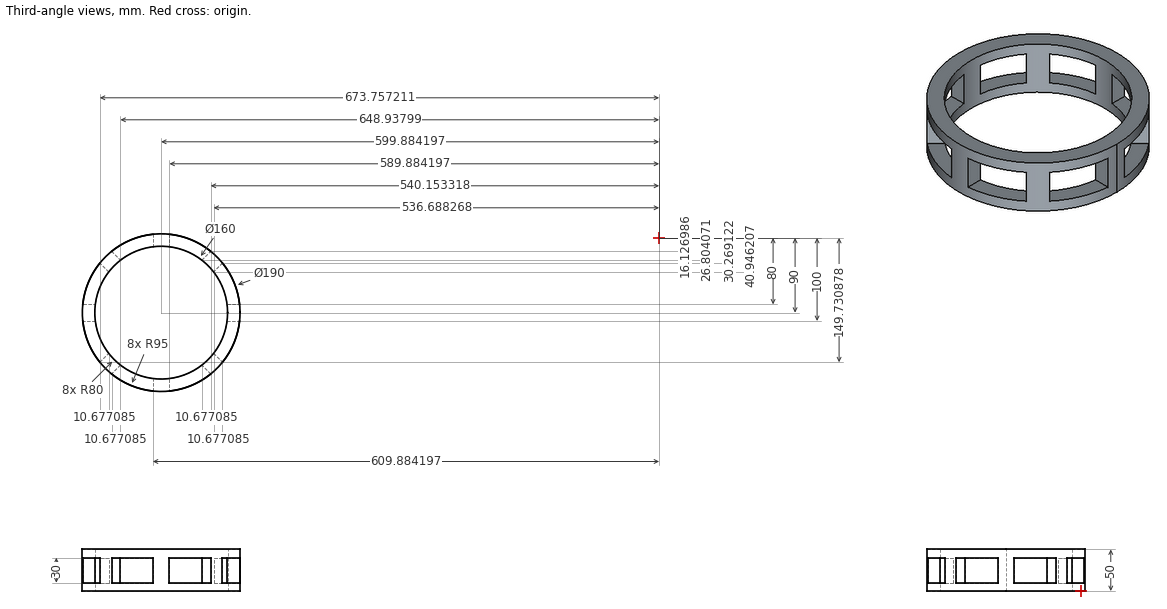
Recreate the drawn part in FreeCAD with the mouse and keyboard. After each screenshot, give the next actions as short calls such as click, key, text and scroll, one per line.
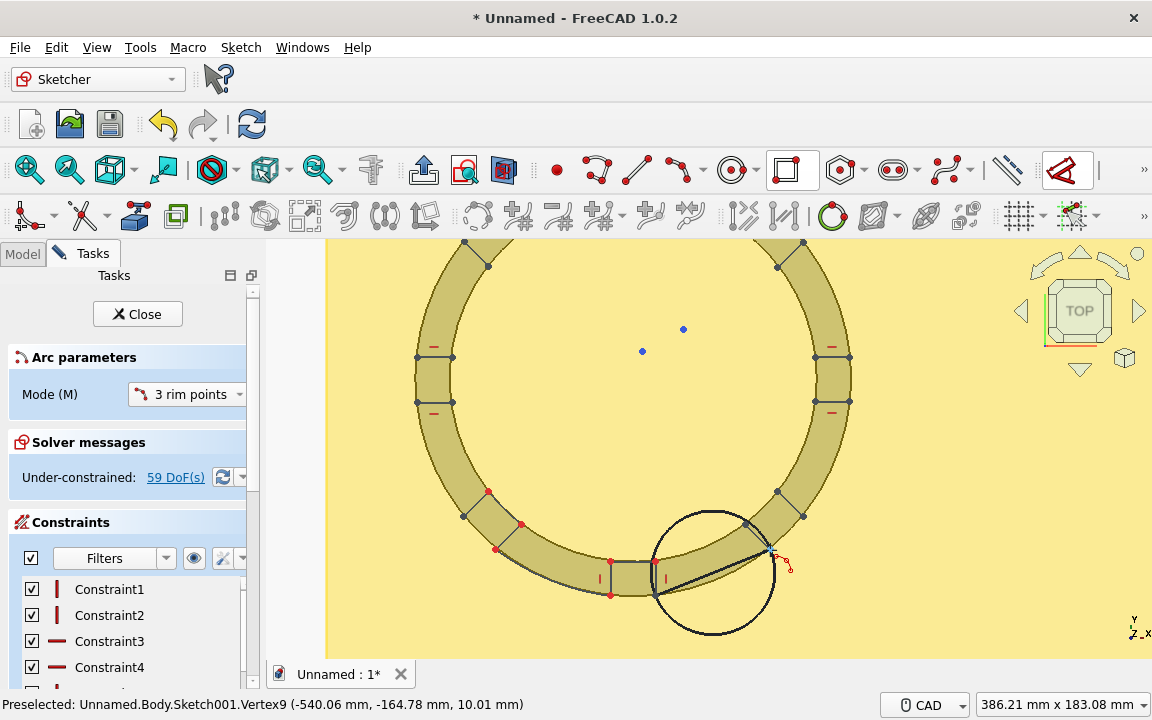
scroll(717, 579, up, 3)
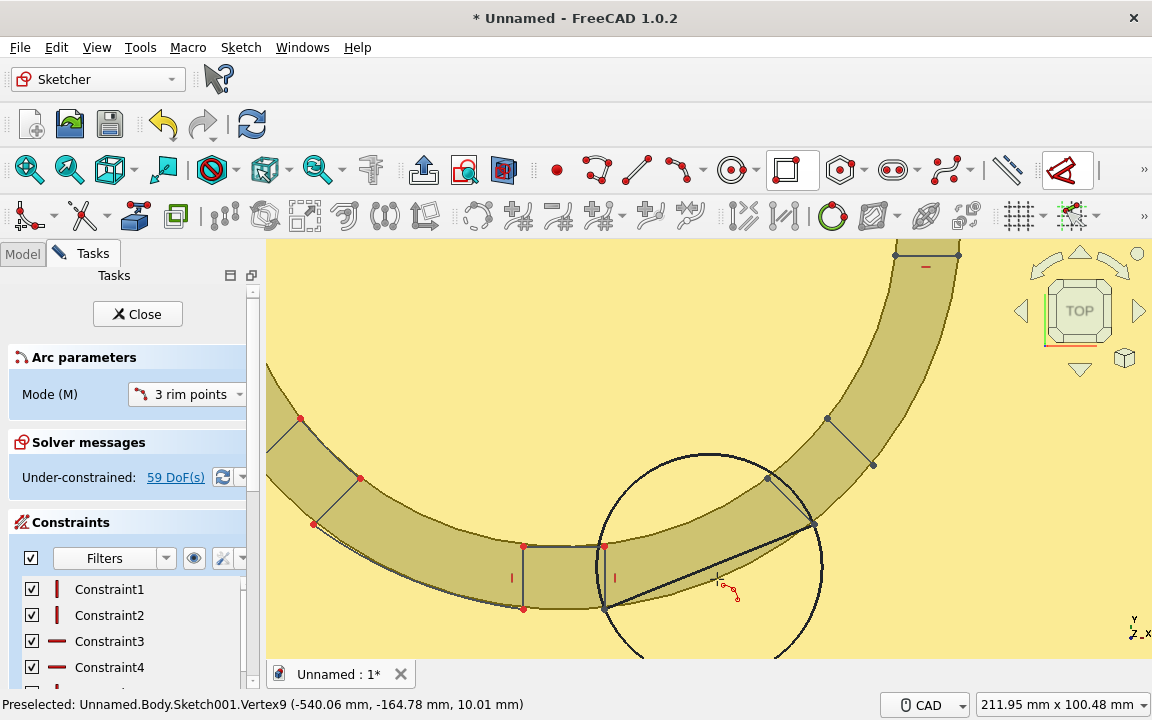
click(716, 579)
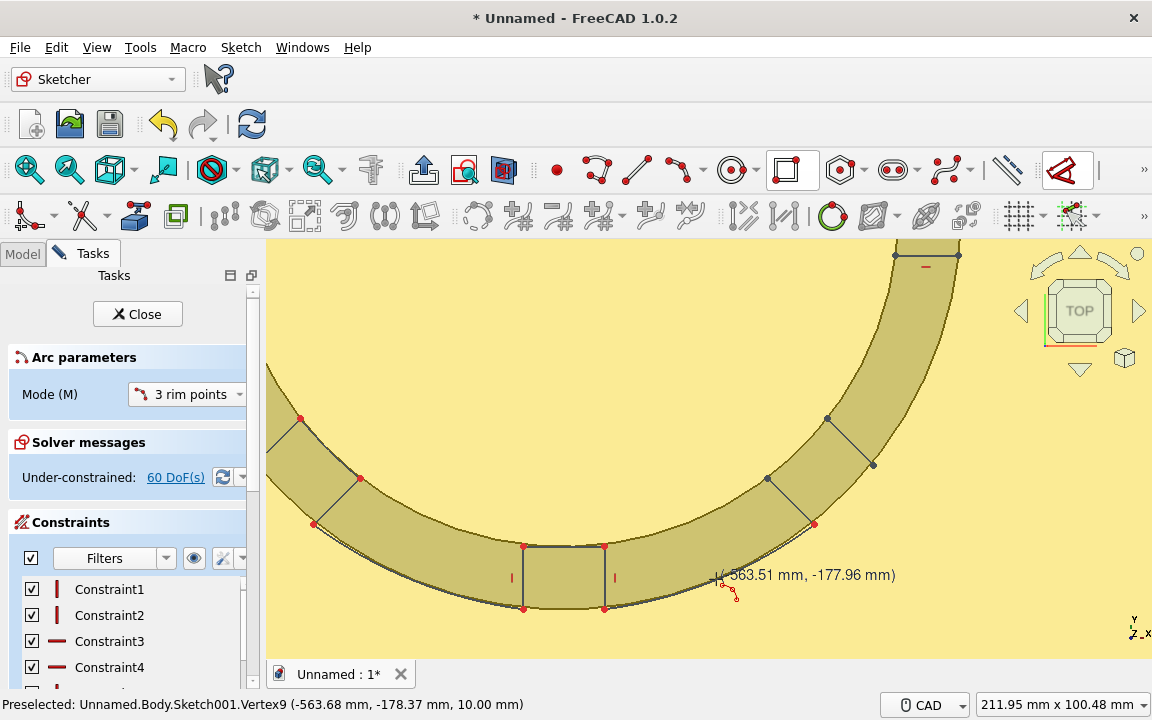
click(768, 479)
click(828, 419)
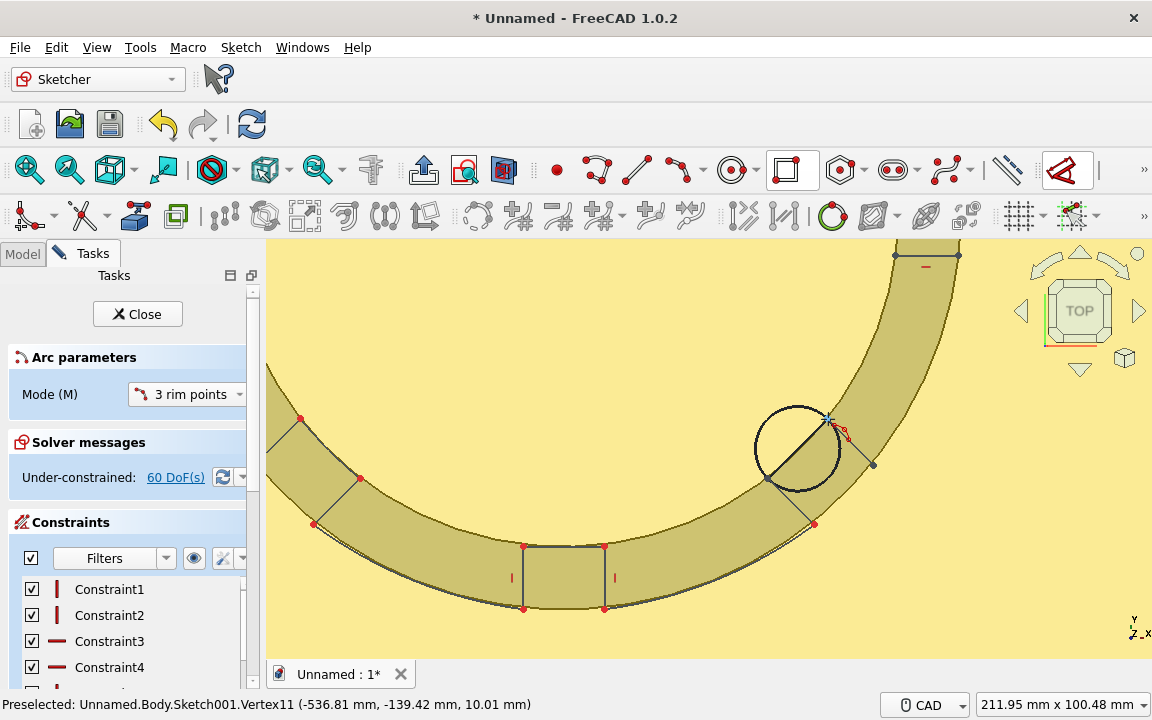
scroll(800, 449, up, 10)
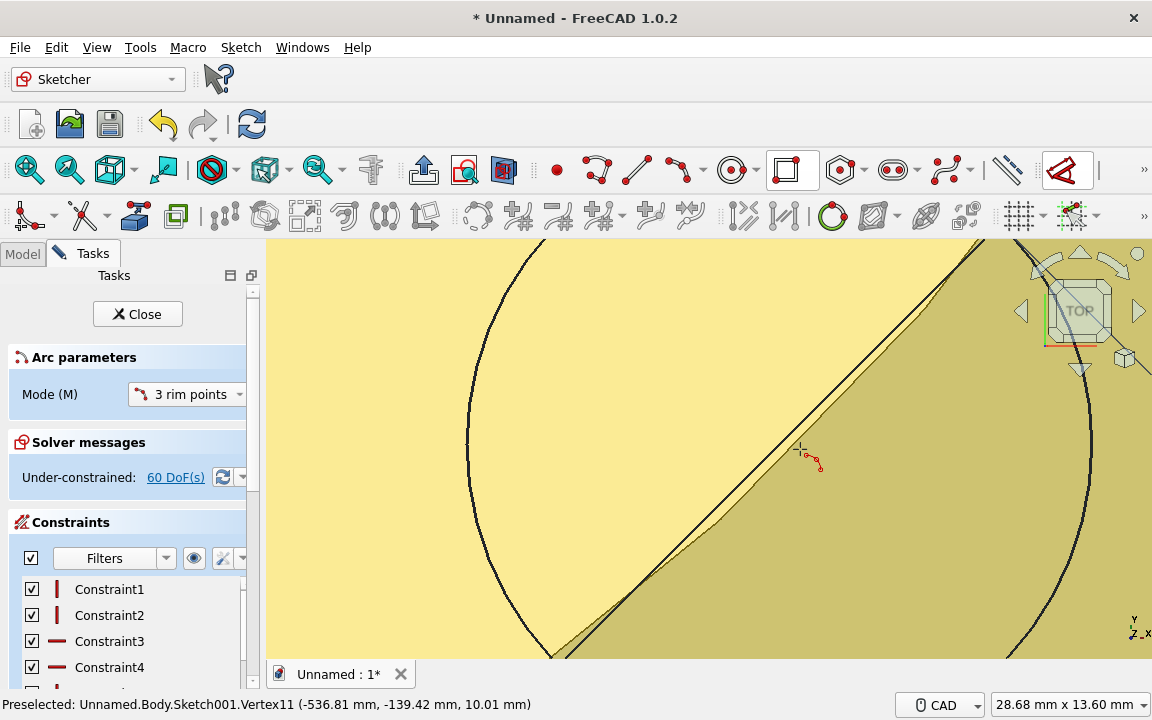
click(799, 444)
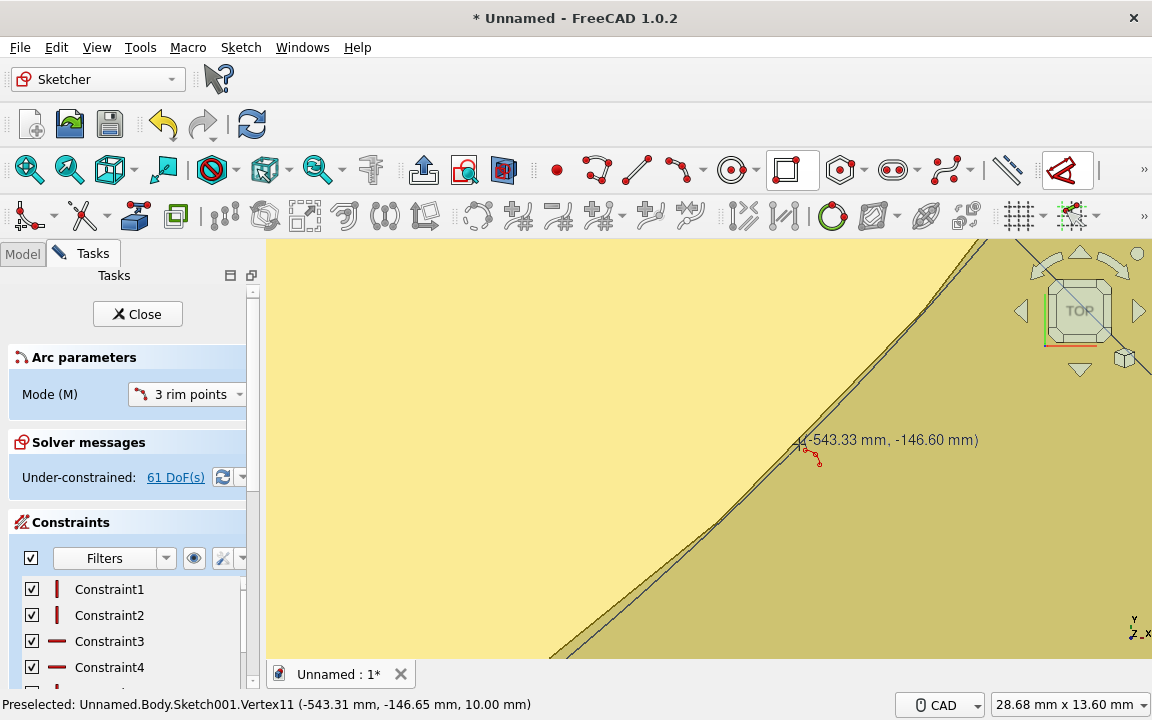
scroll(724, 541, down, 15)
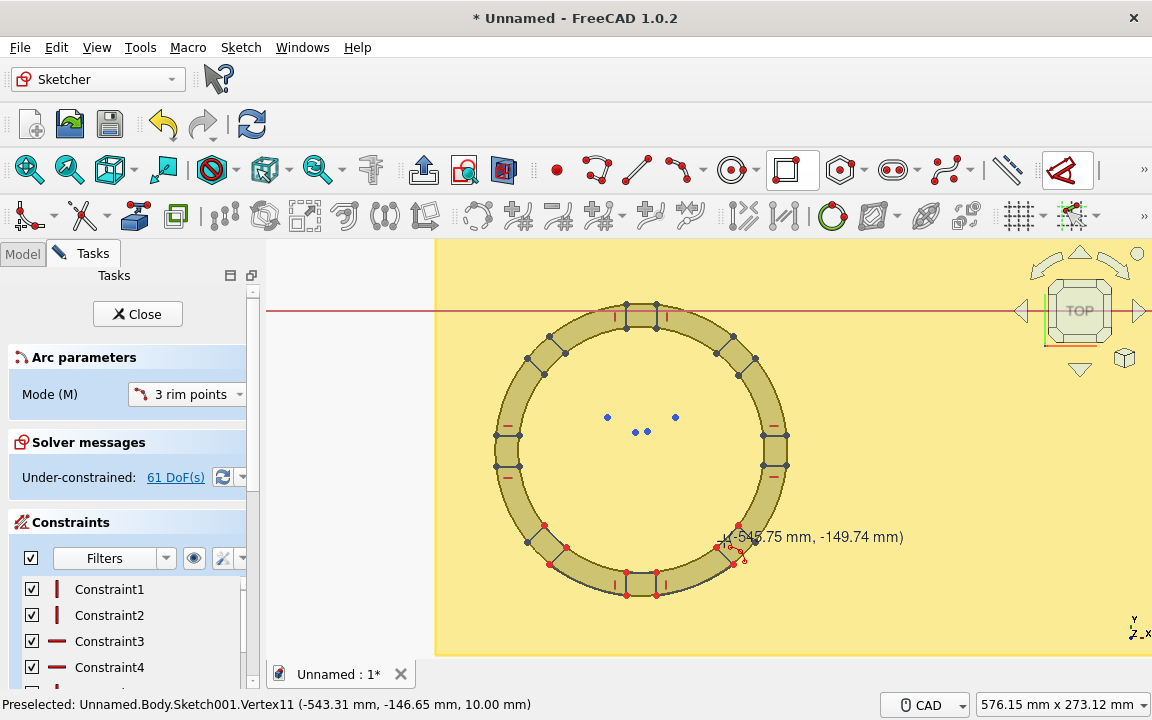
scroll(755, 542, up, 2)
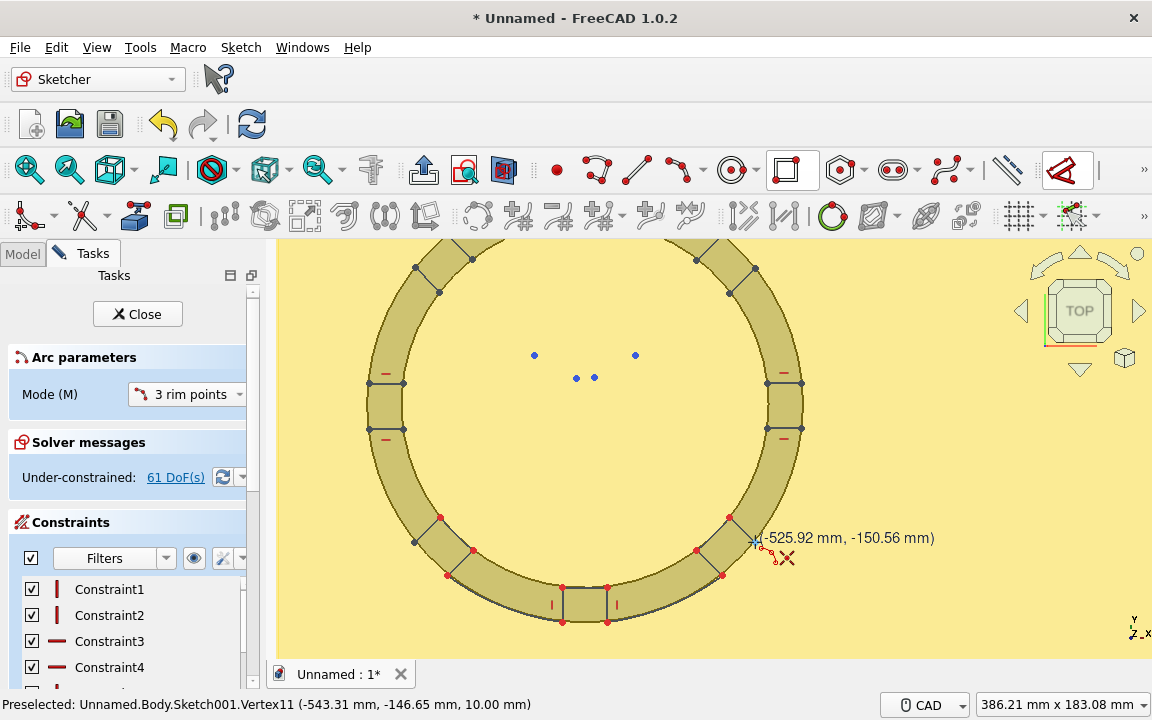
click(755, 543)
click(801, 428)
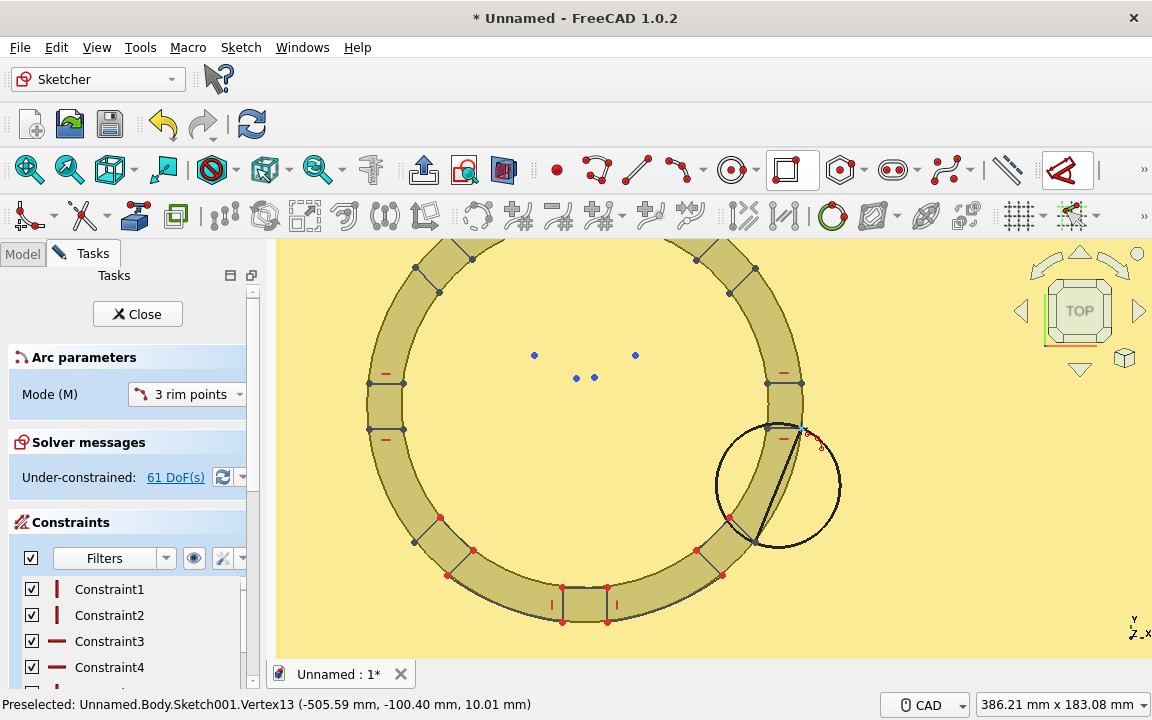
scroll(786, 488, up, 3)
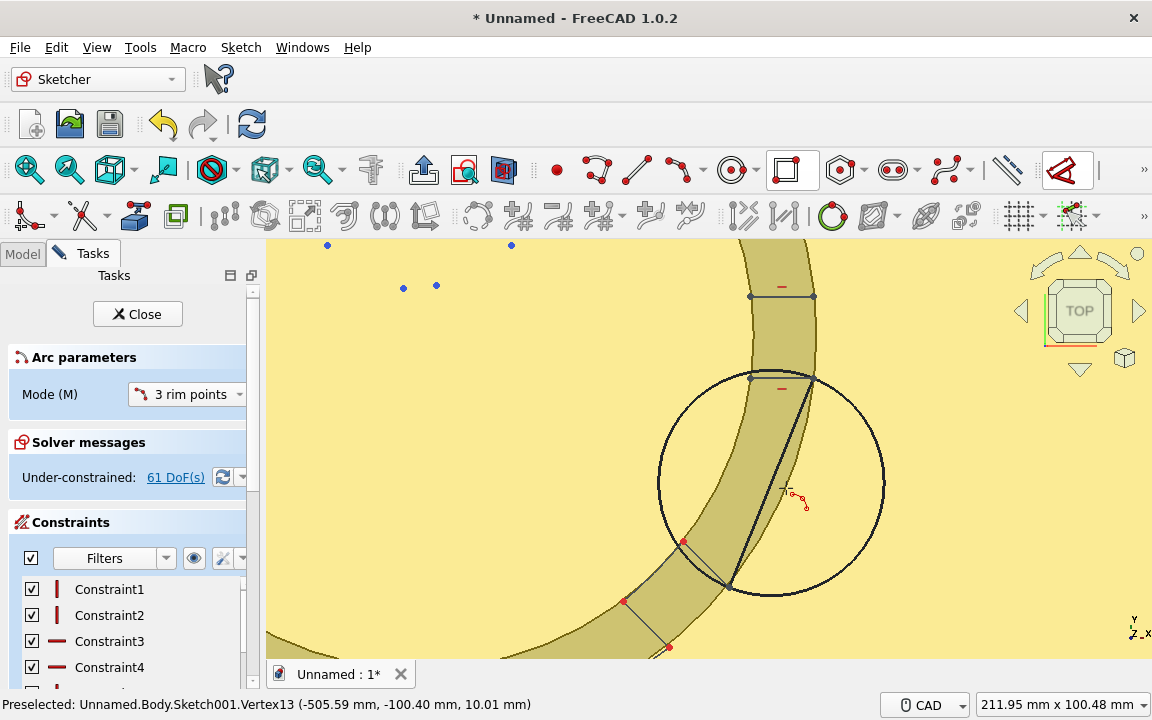
click(786, 487)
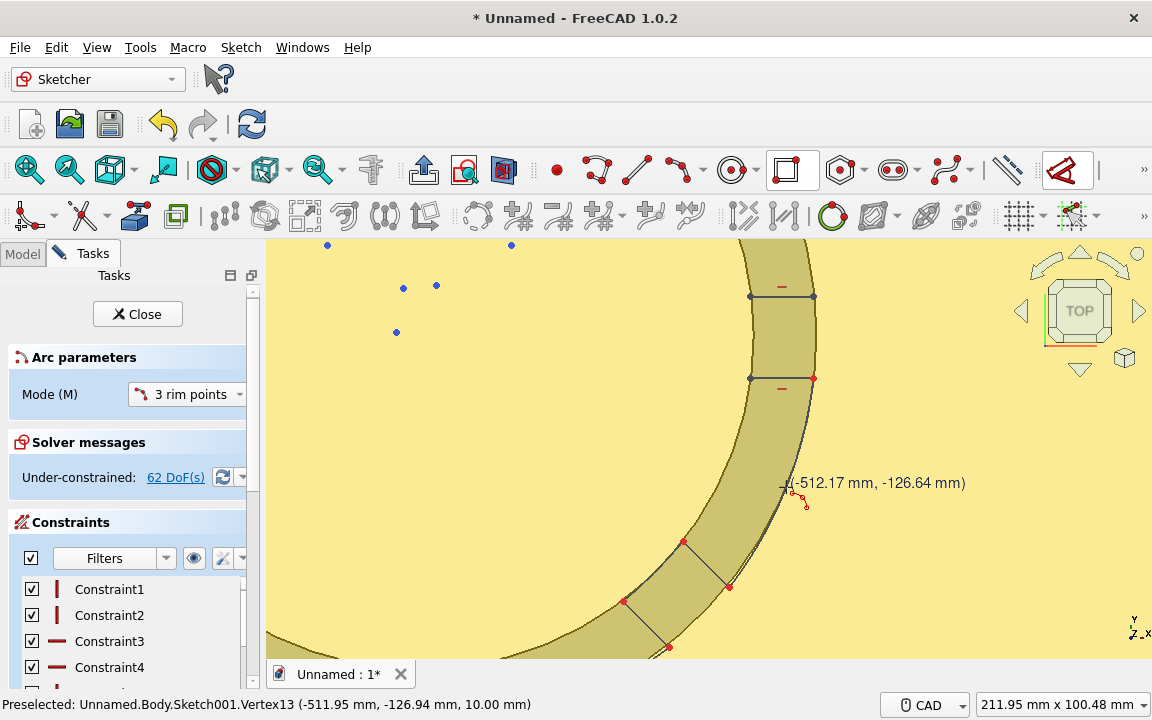
click(751, 378)
click(751, 297)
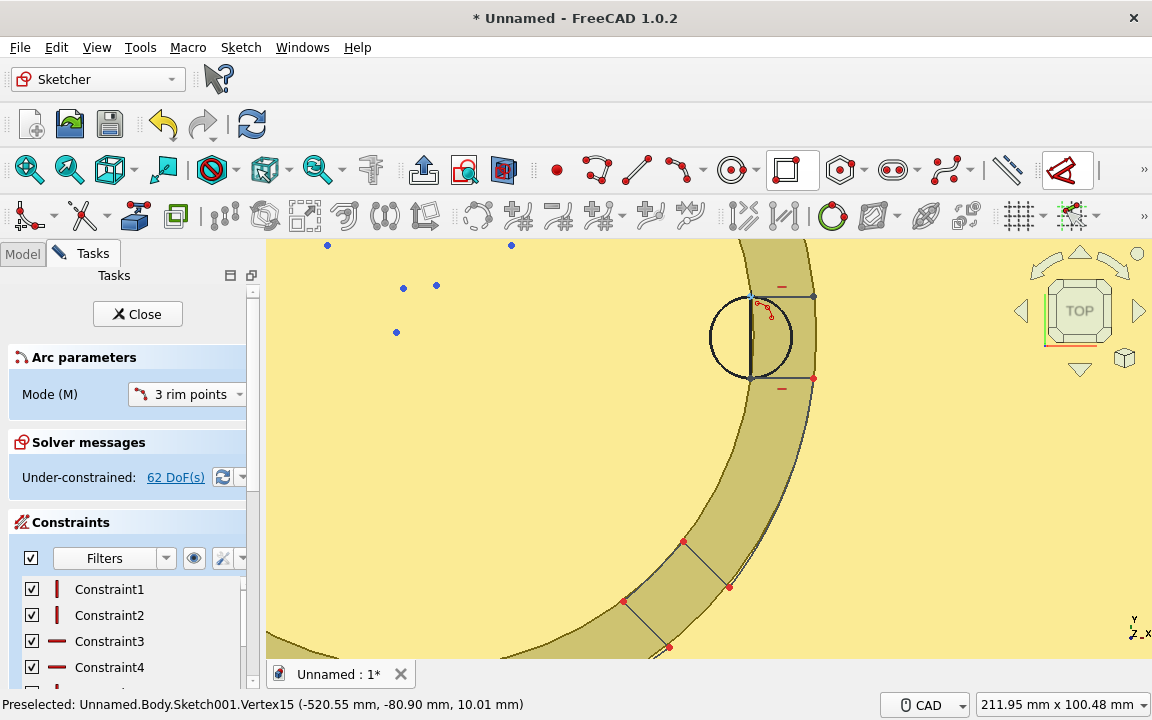
scroll(754, 335, up, 10)